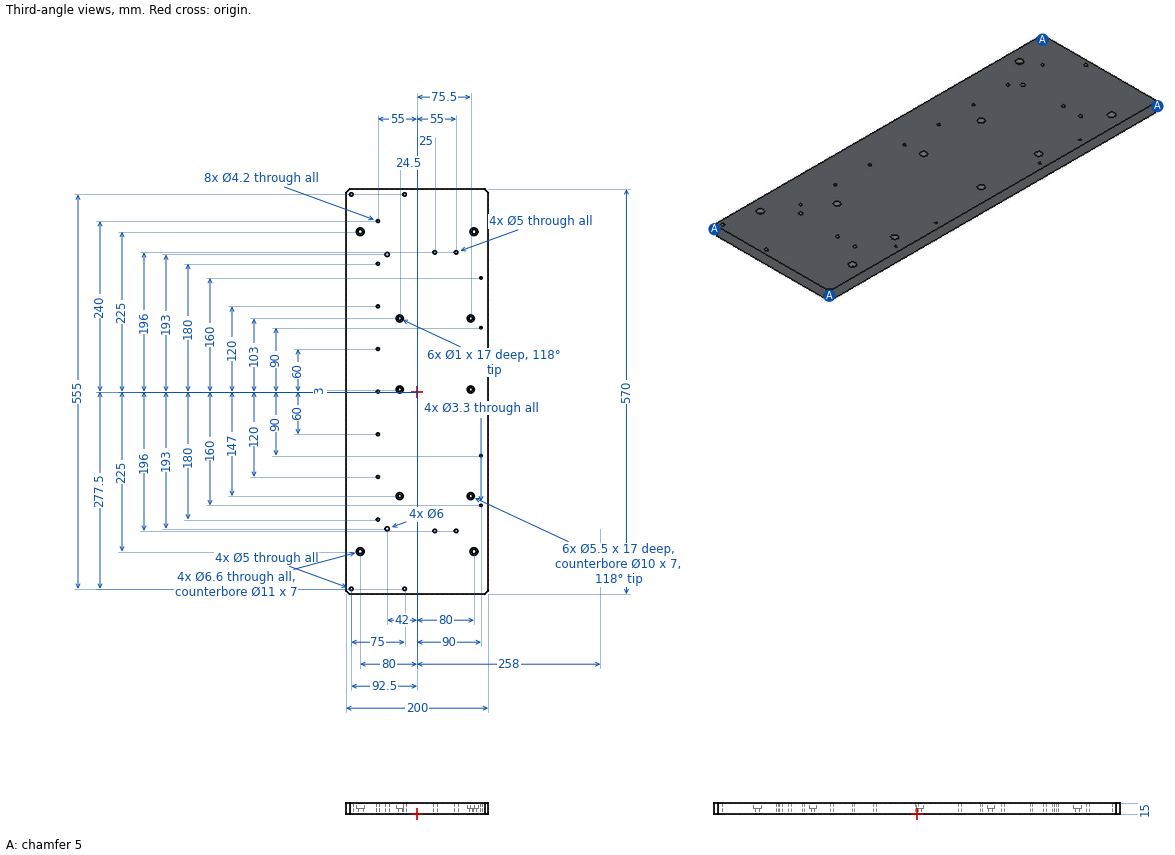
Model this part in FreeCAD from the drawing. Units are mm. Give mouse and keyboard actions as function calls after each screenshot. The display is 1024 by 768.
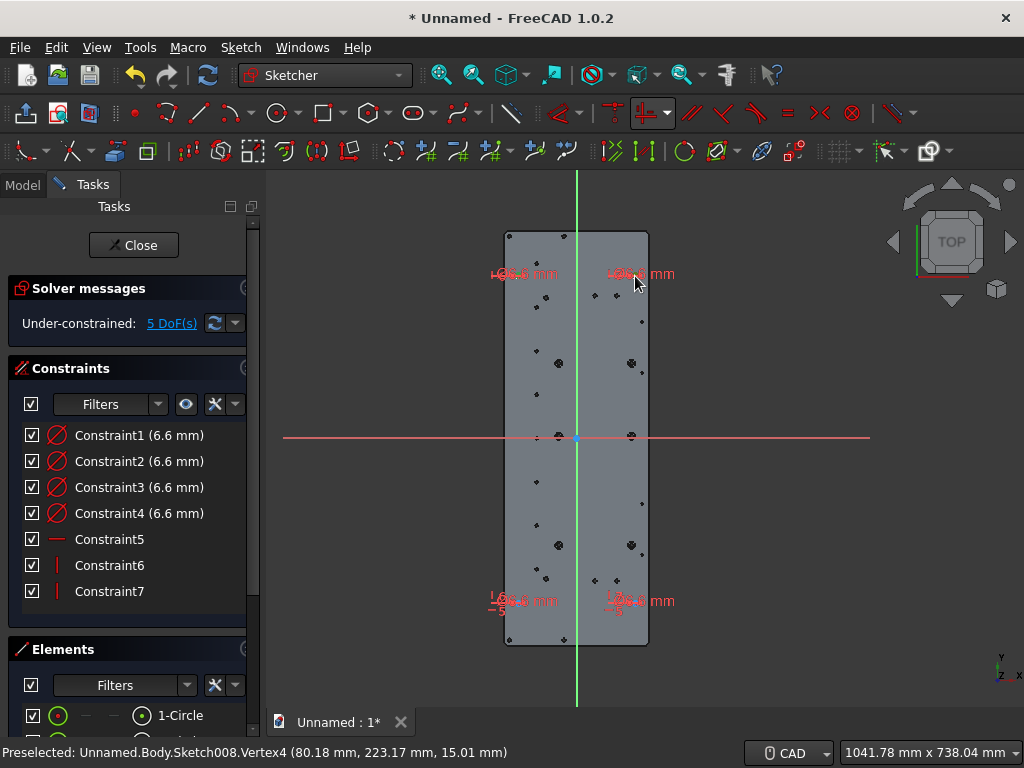
key(h)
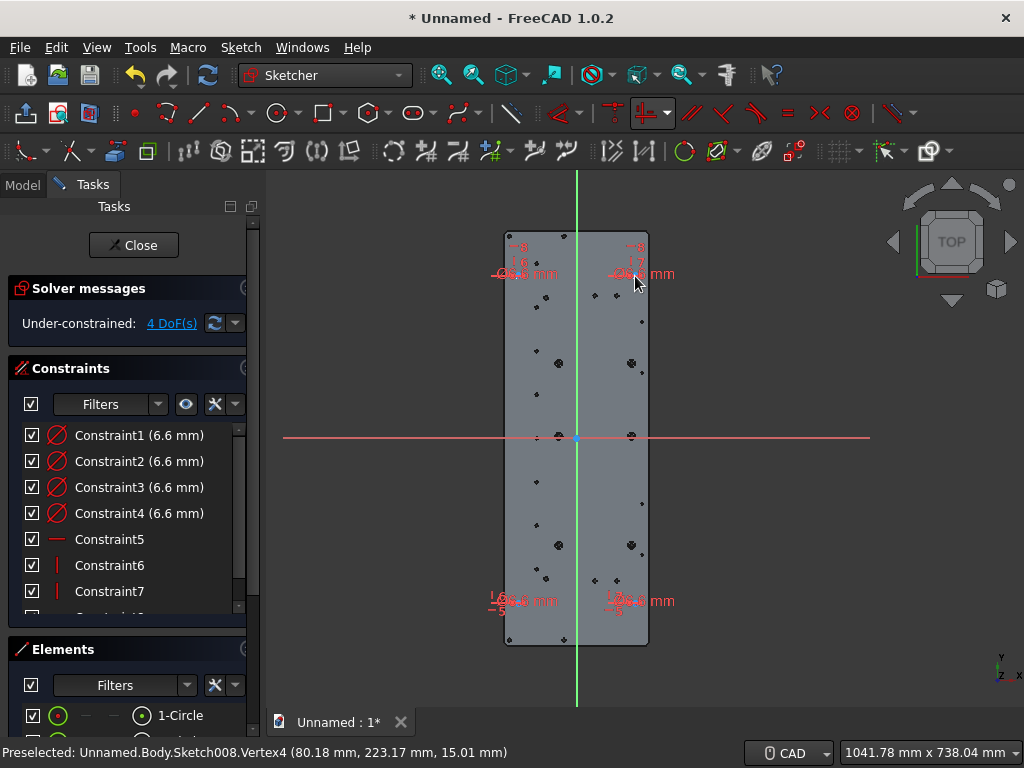
click(558, 114)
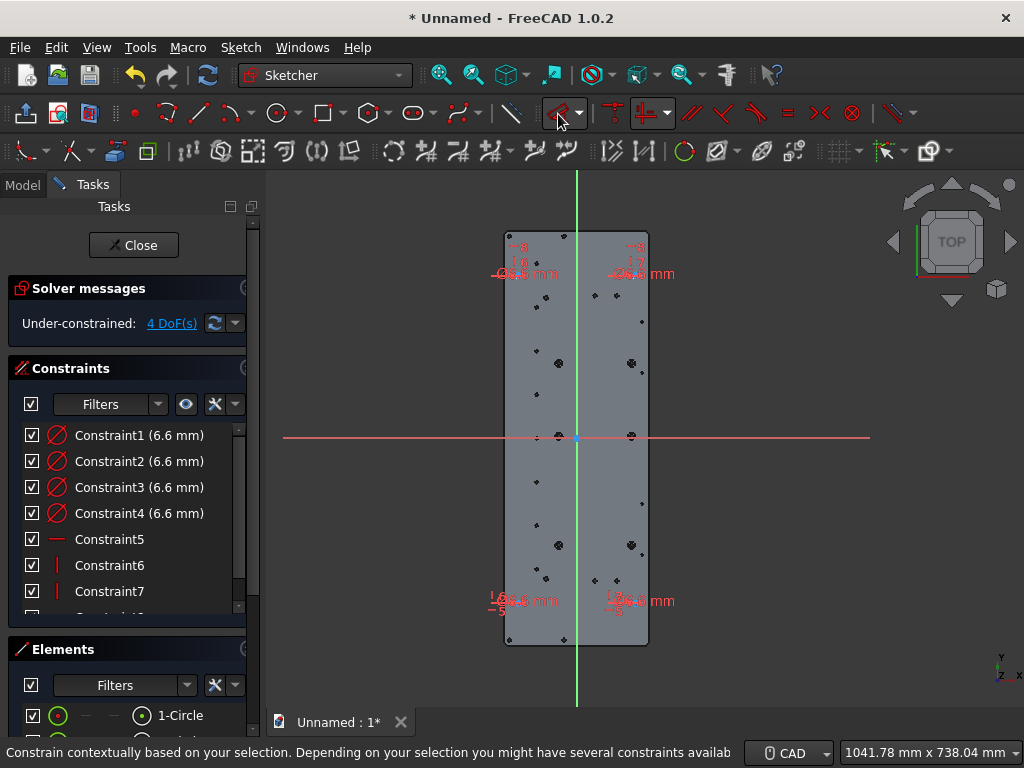
click(518, 603)
click(547, 637)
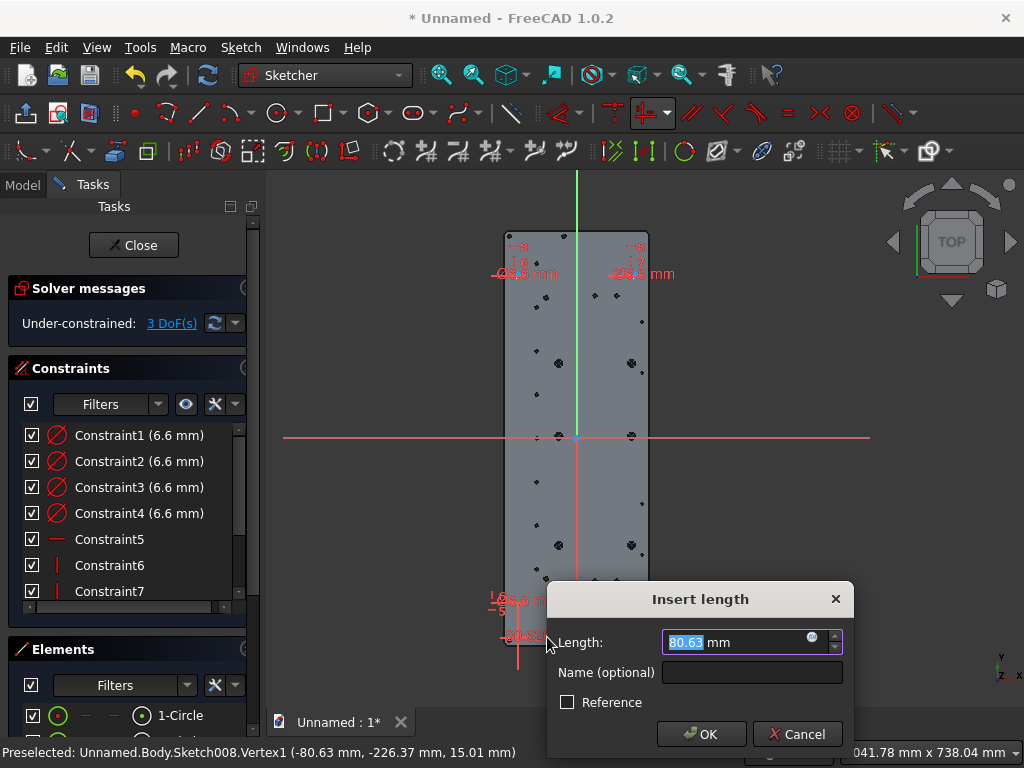
text(80)
key(Return)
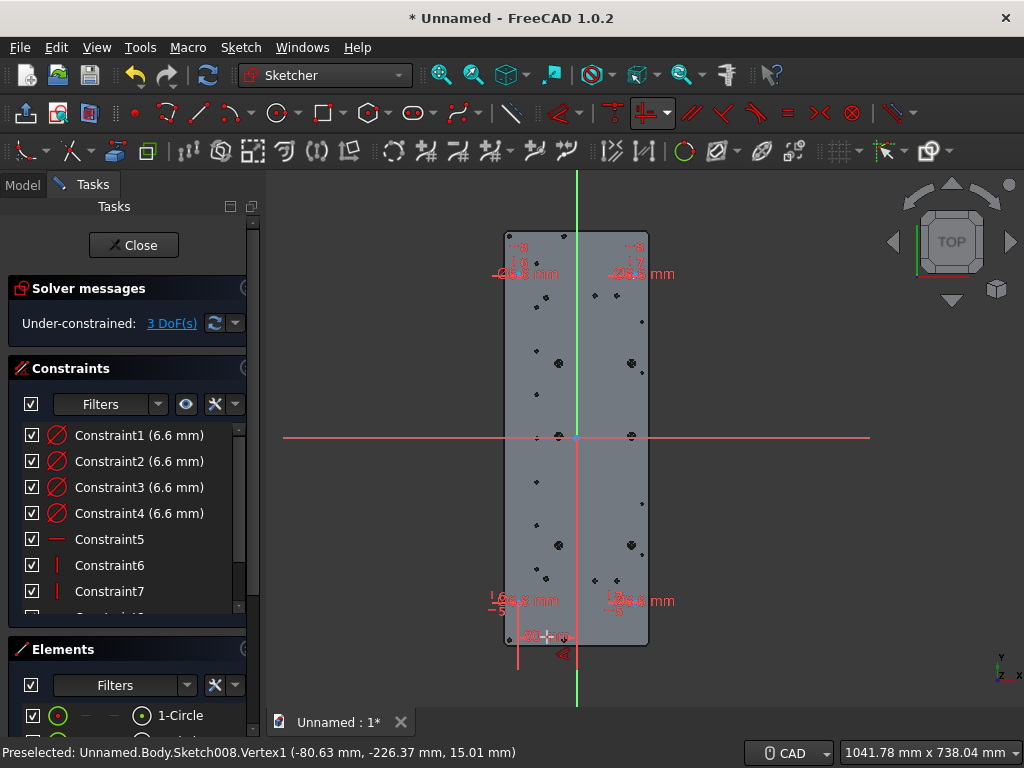
click(635, 603)
click(619, 637)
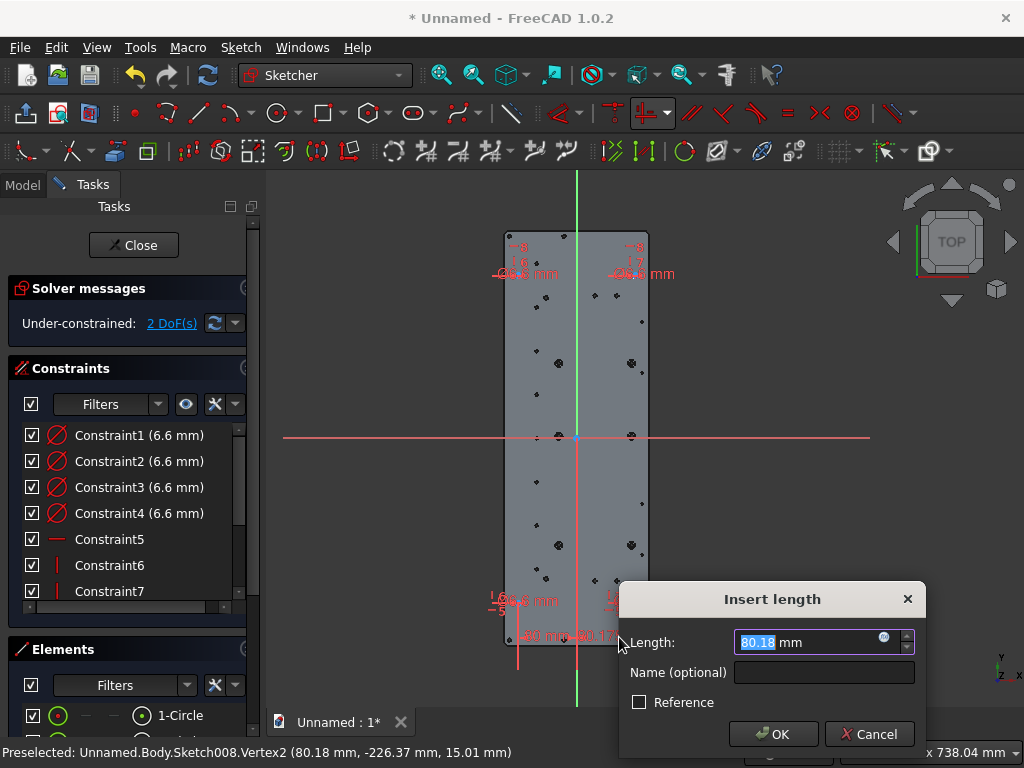
text(80)
key(Return)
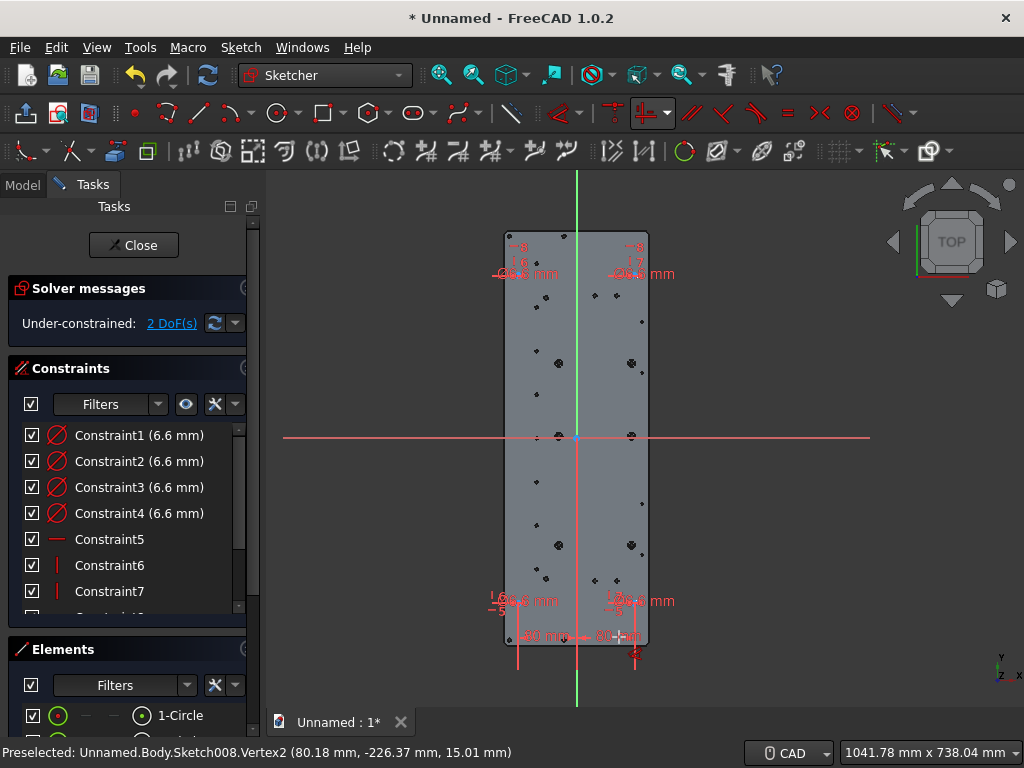
click(518, 603)
click(484, 521)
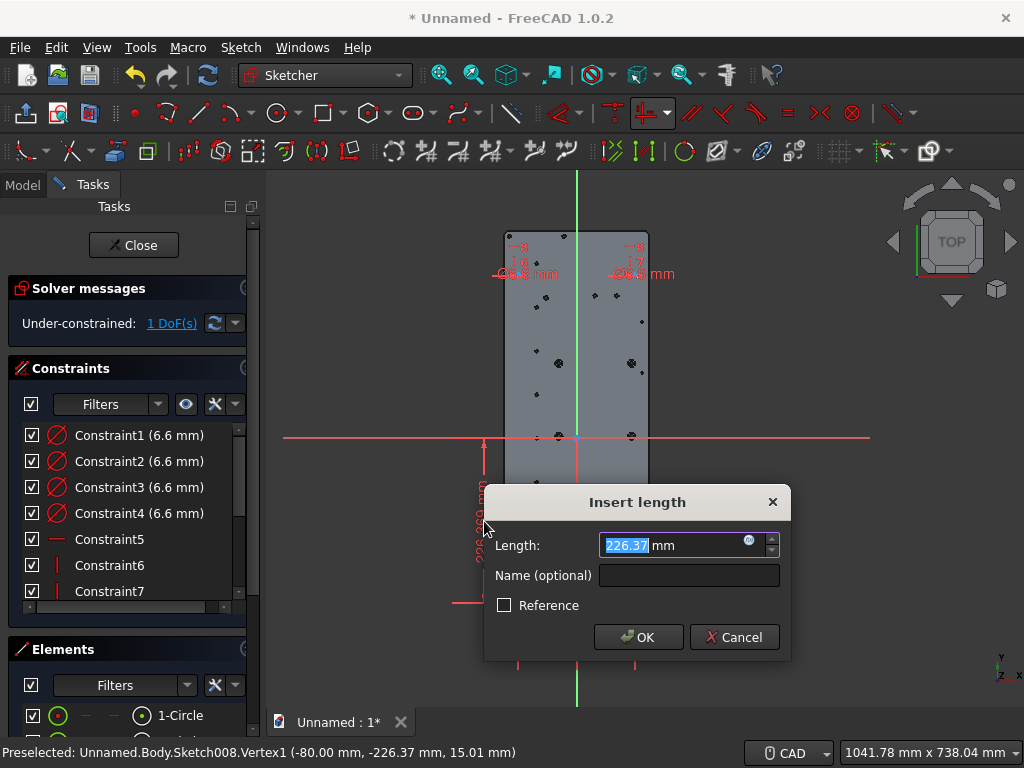
text(225)
key(Return)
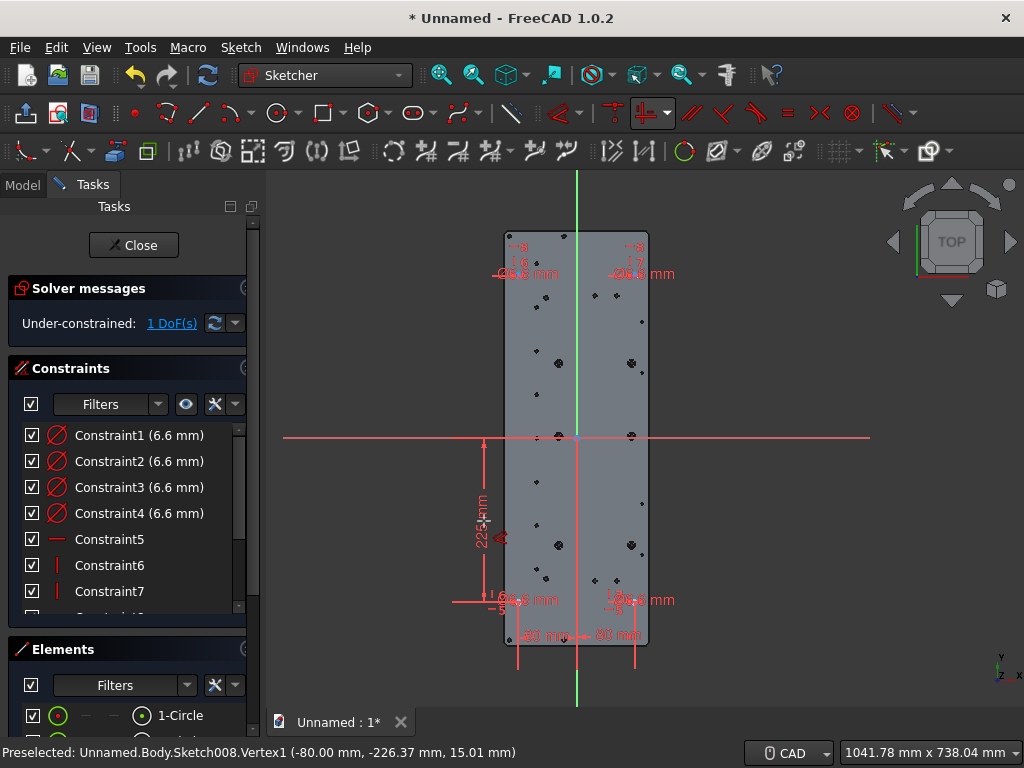
click(518, 276)
click(484, 357)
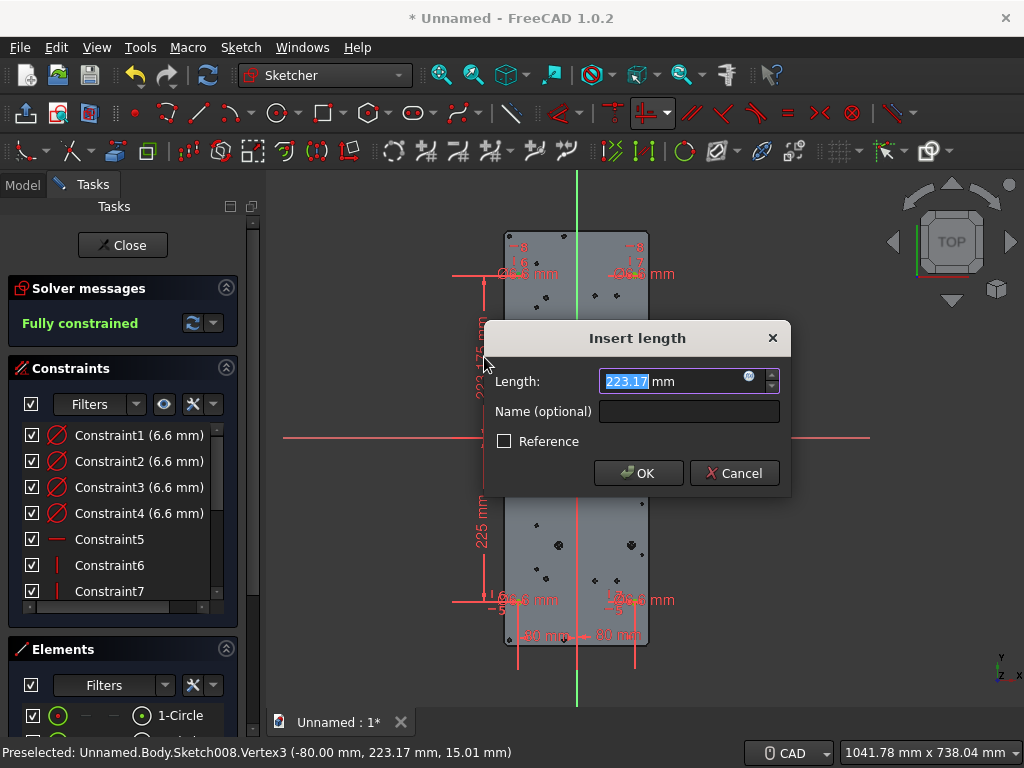
text(225)
key(Return)
key(Escape)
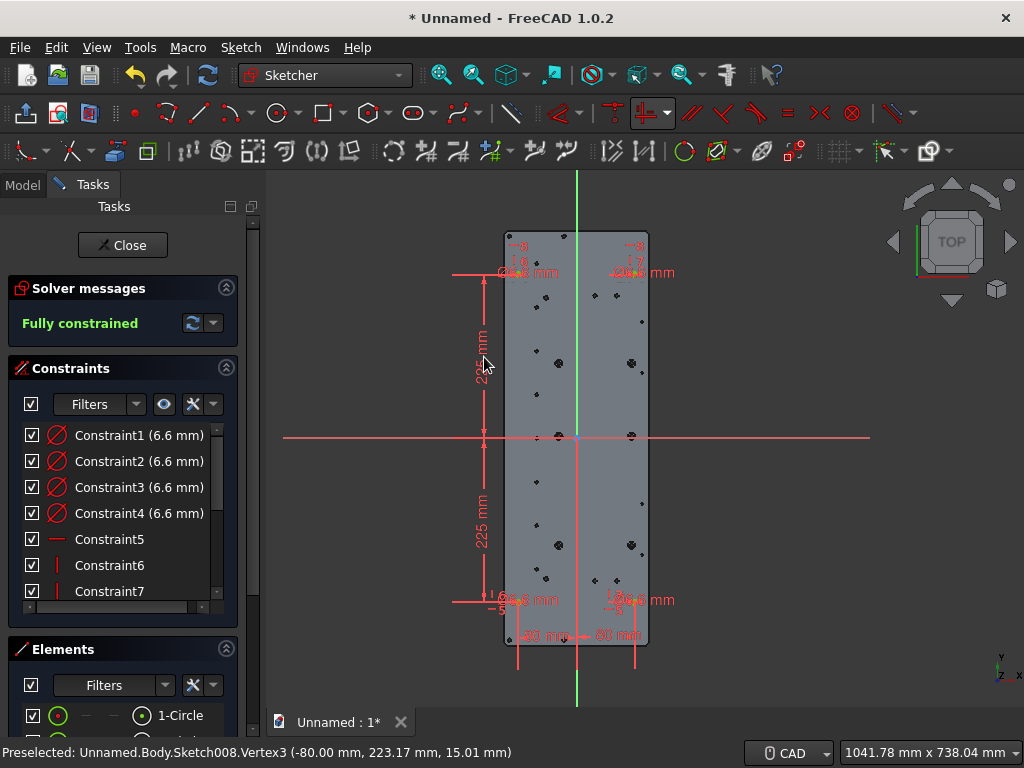
click(123, 245)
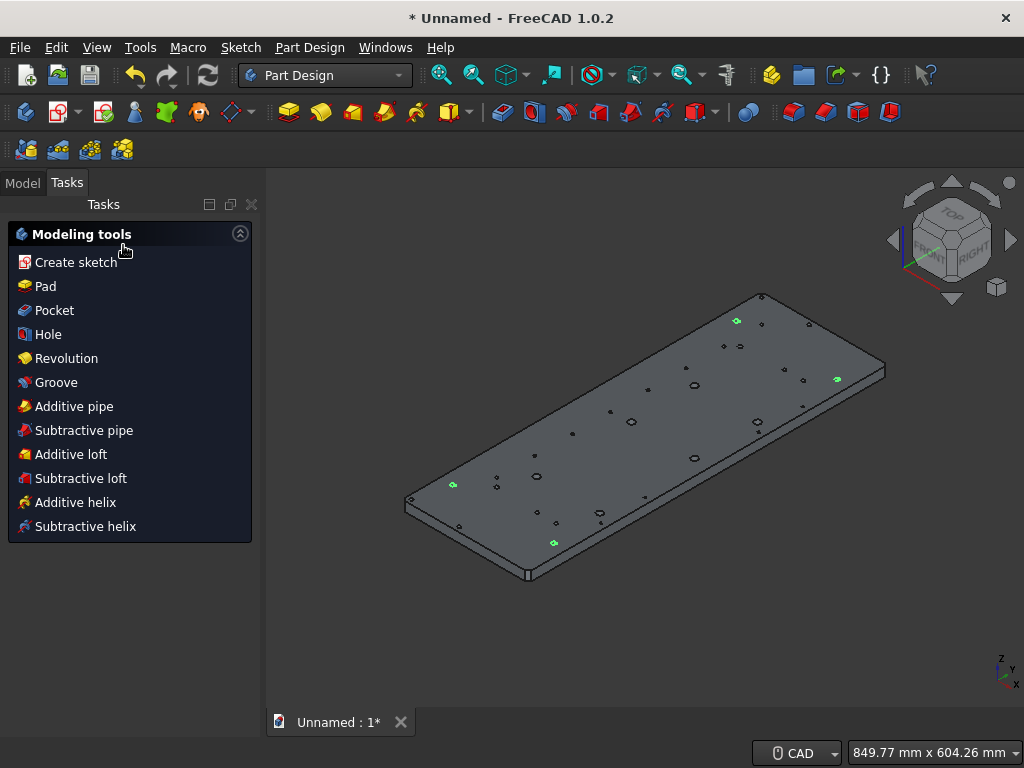
click(536, 112)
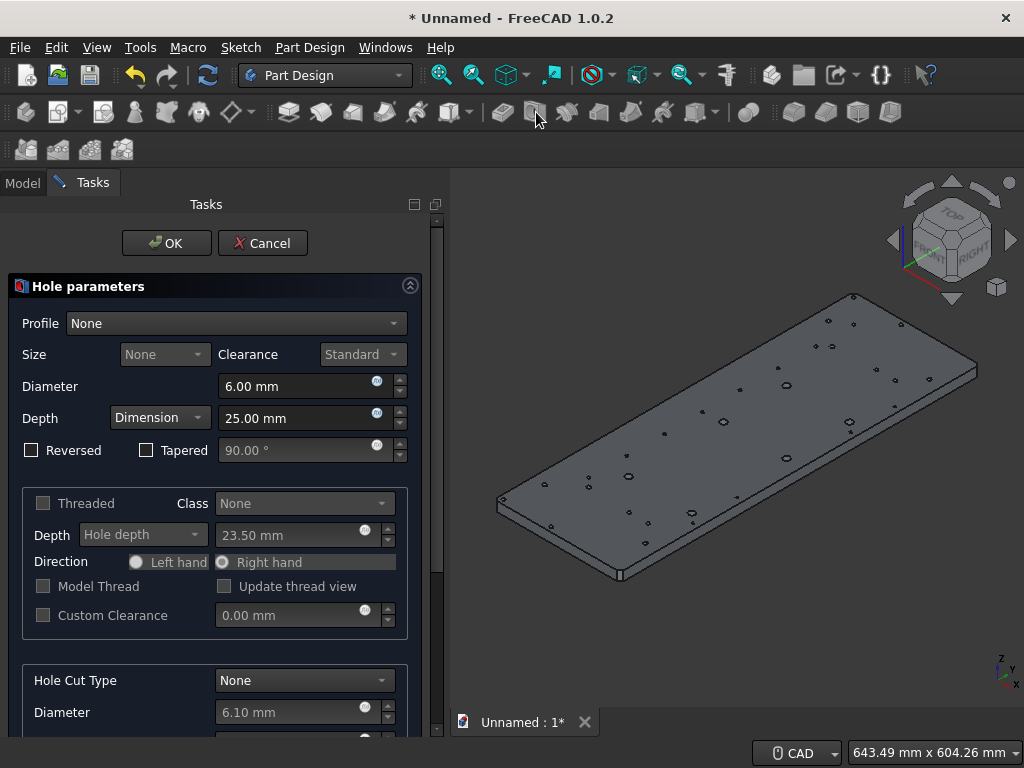
triple_click(305, 386)